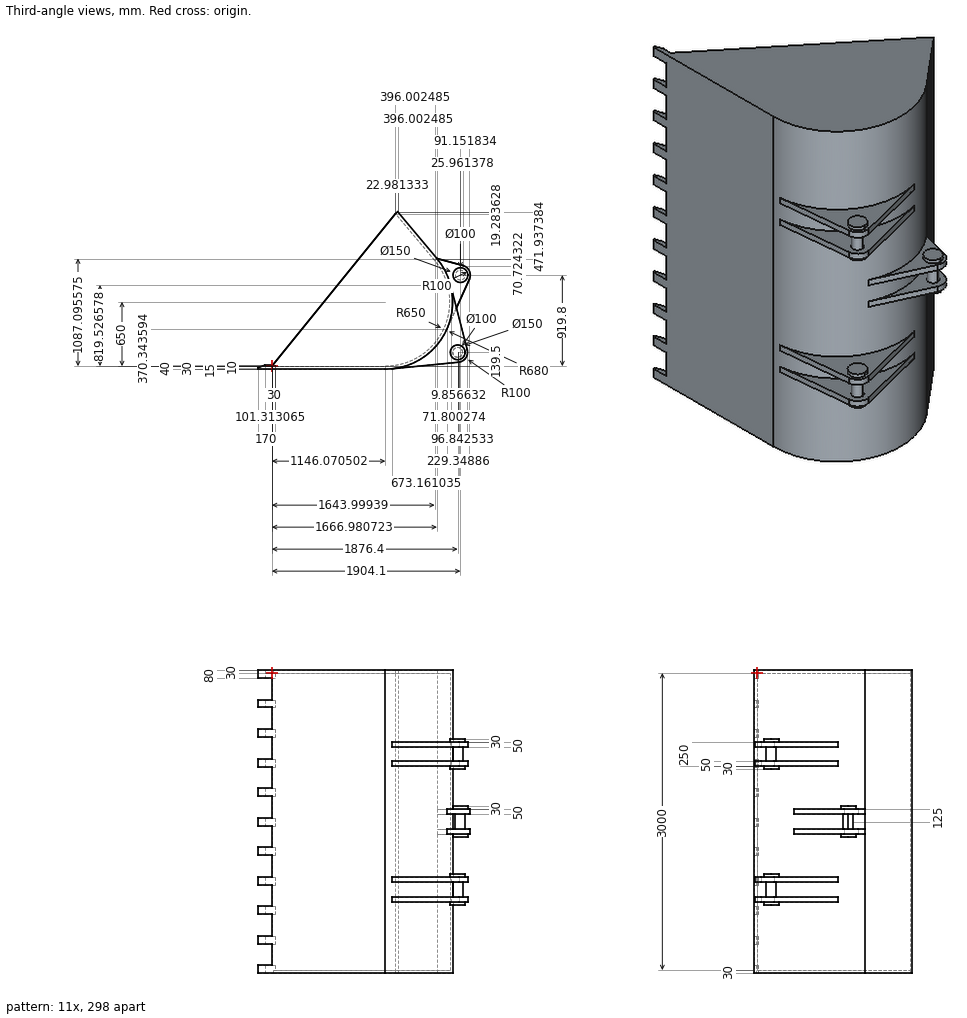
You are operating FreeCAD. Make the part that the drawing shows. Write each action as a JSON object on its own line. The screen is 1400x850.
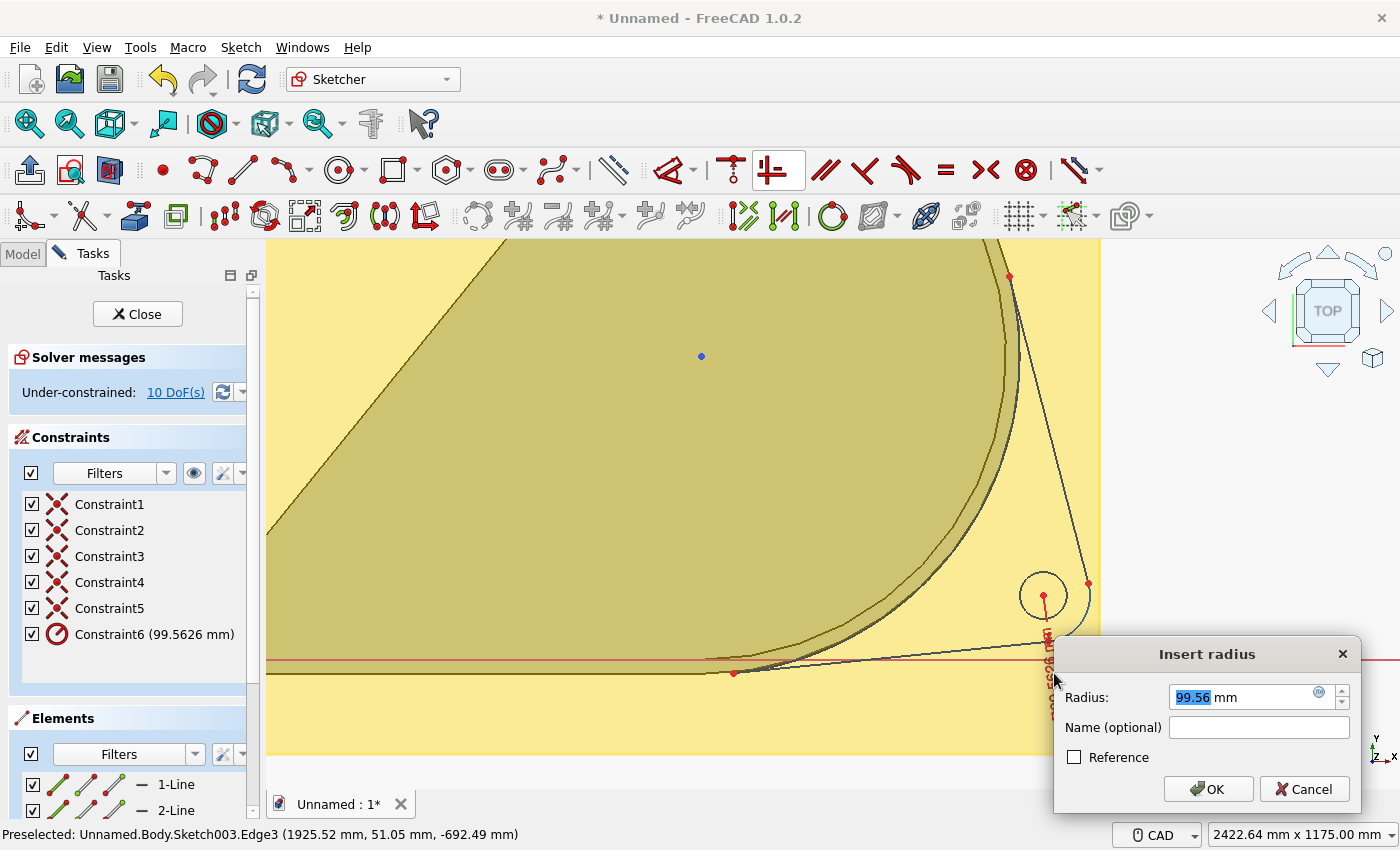
{"action": "type", "text": "100"}
{"action": "key", "text": "Return"}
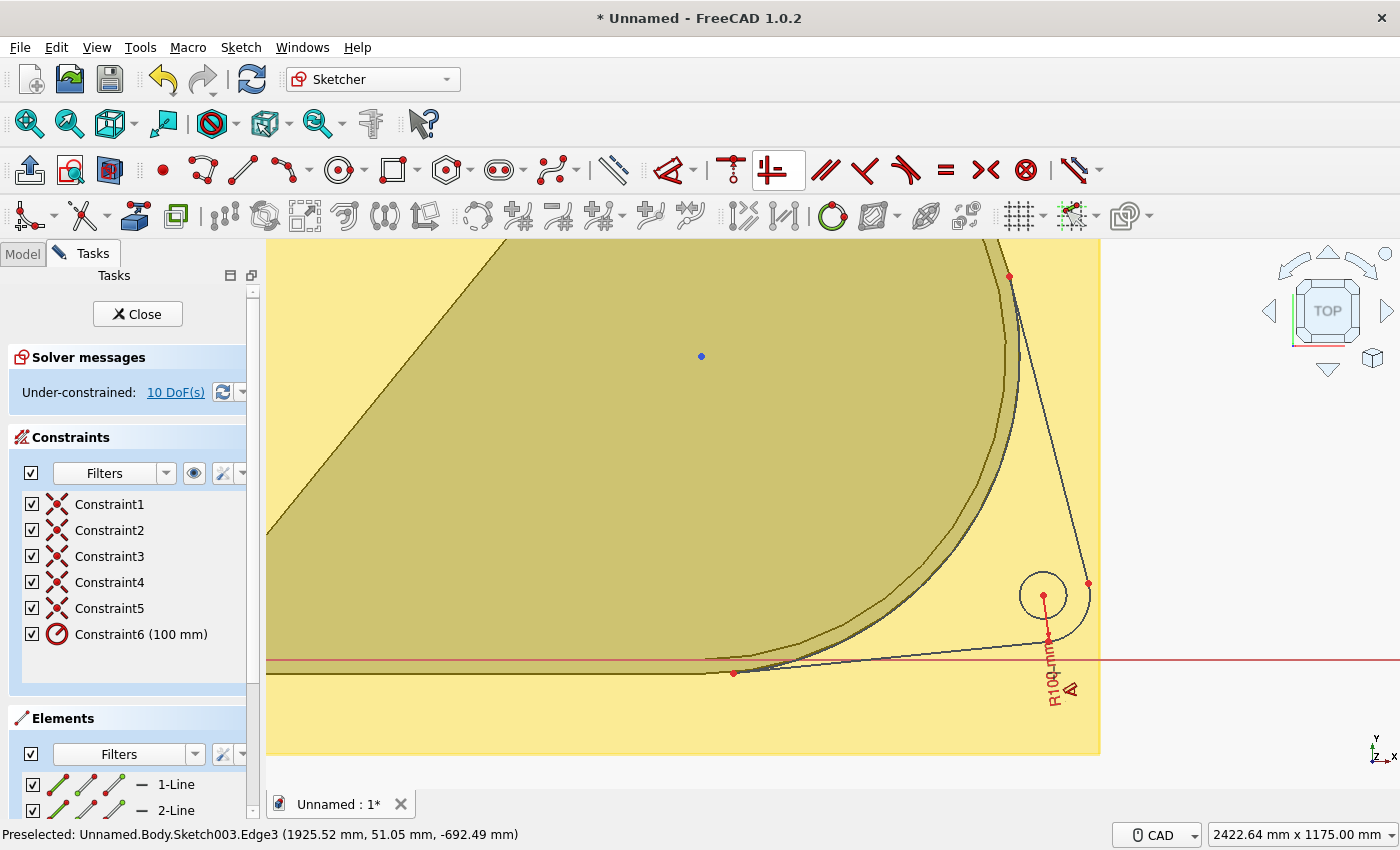
{"action": "left_click", "coordinate": [886, 616]}
{"action": "left_click", "coordinate": [905, 642]}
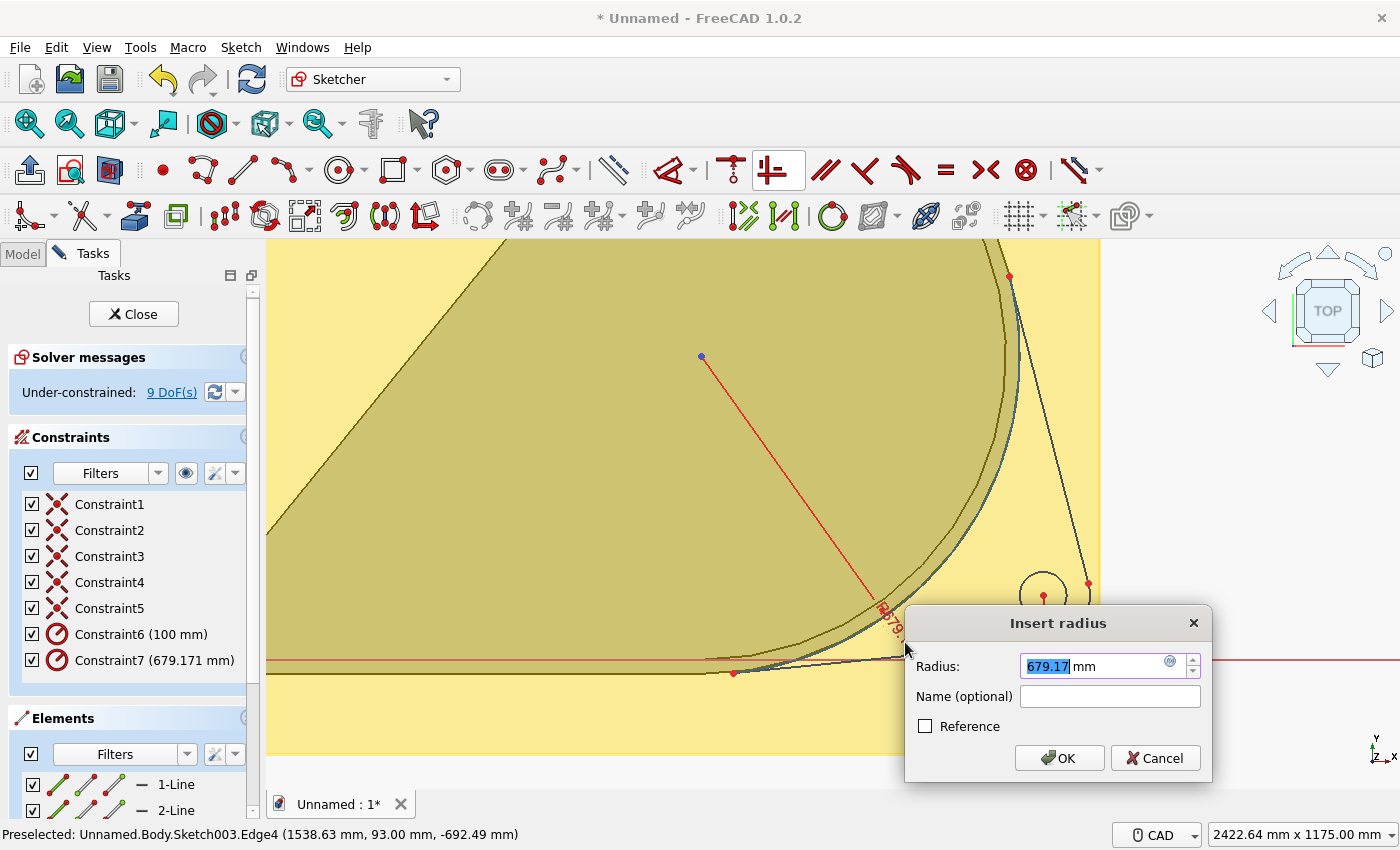
{"action": "type", "text": "680"}
{"action": "key", "text": "Return"}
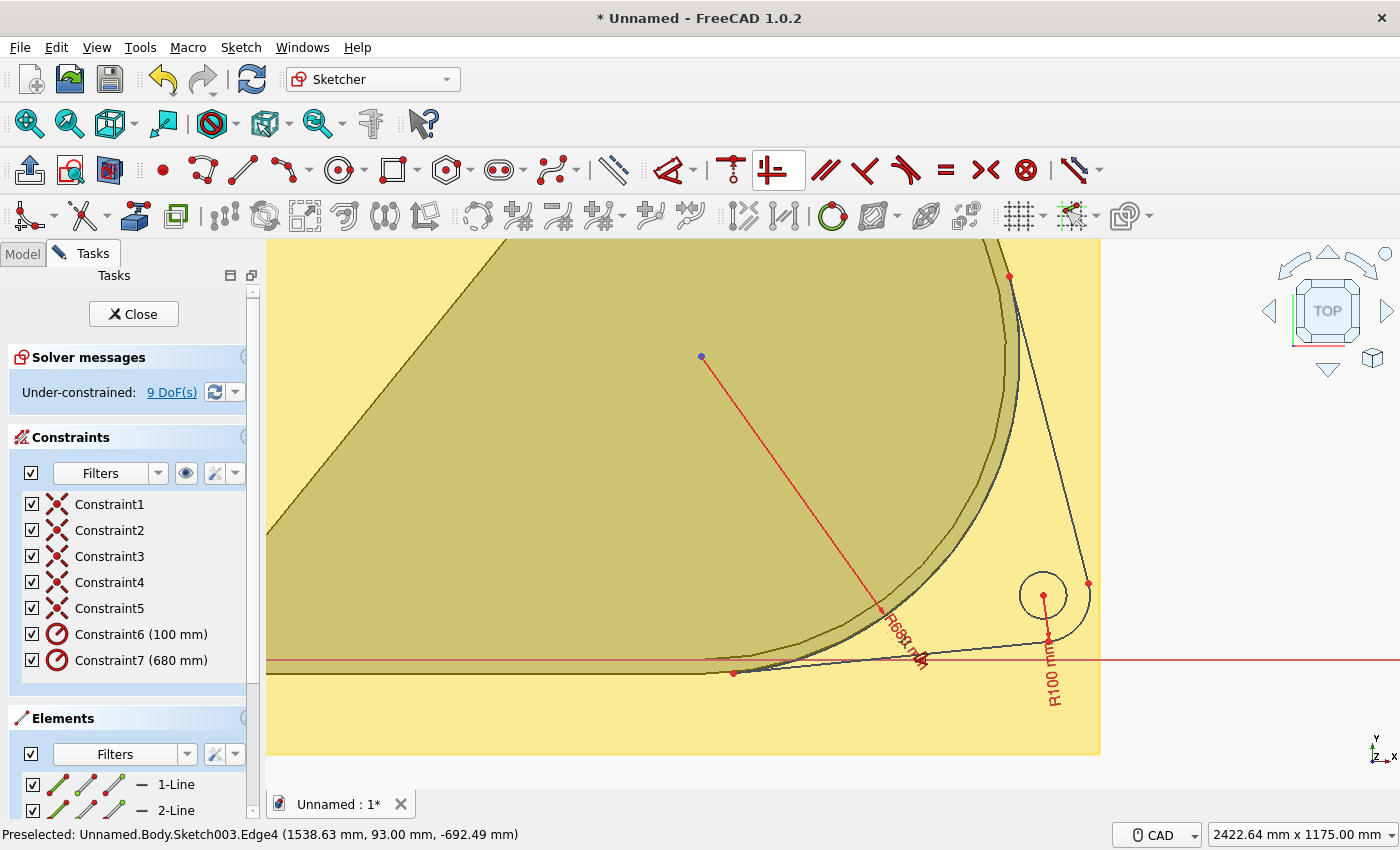
{"action": "left_click", "coordinate": [1060, 579]}
{"action": "left_click", "coordinate": [1060, 542]}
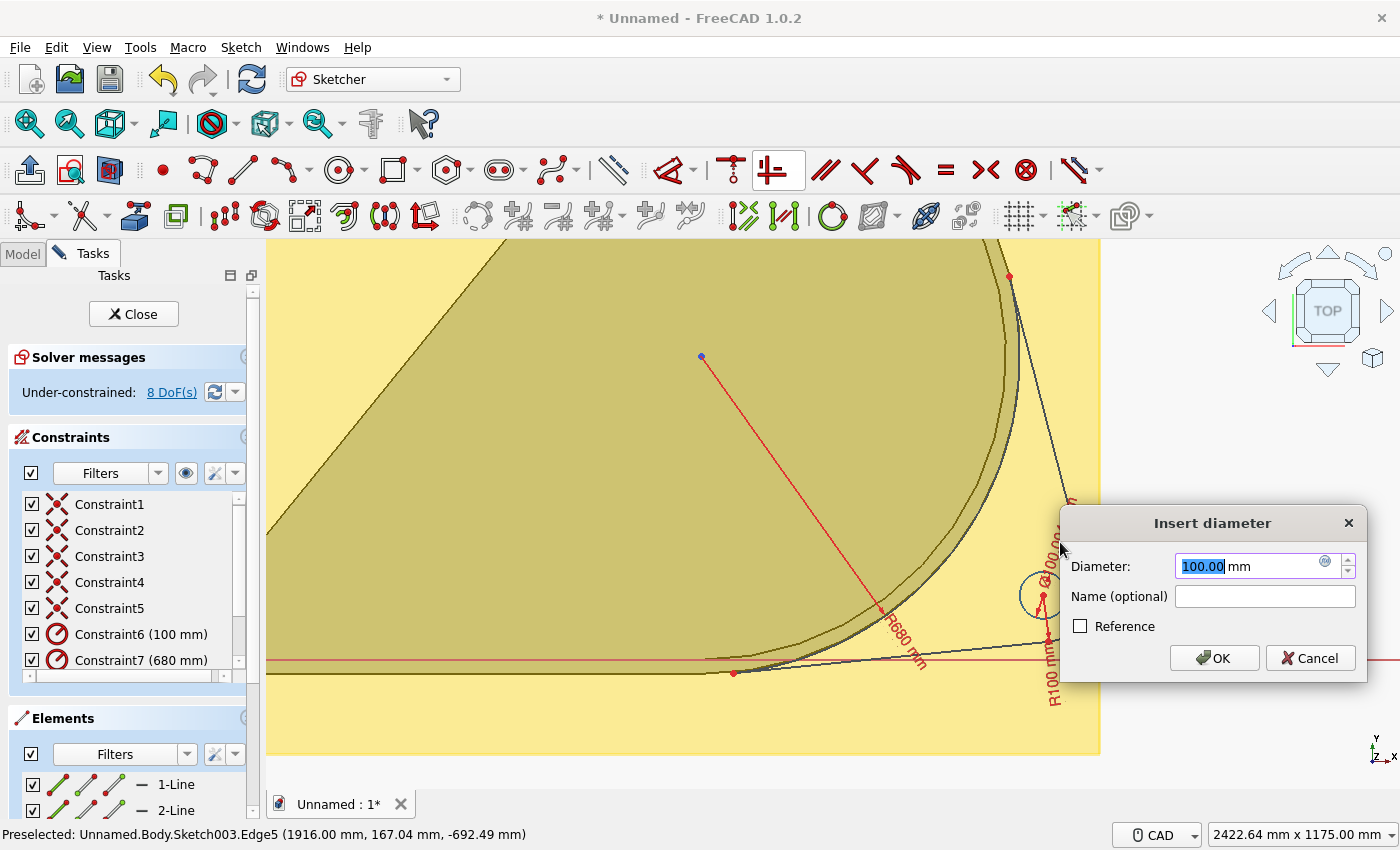
{"action": "type", "text": "100"}
{"action": "key", "text": "Return"}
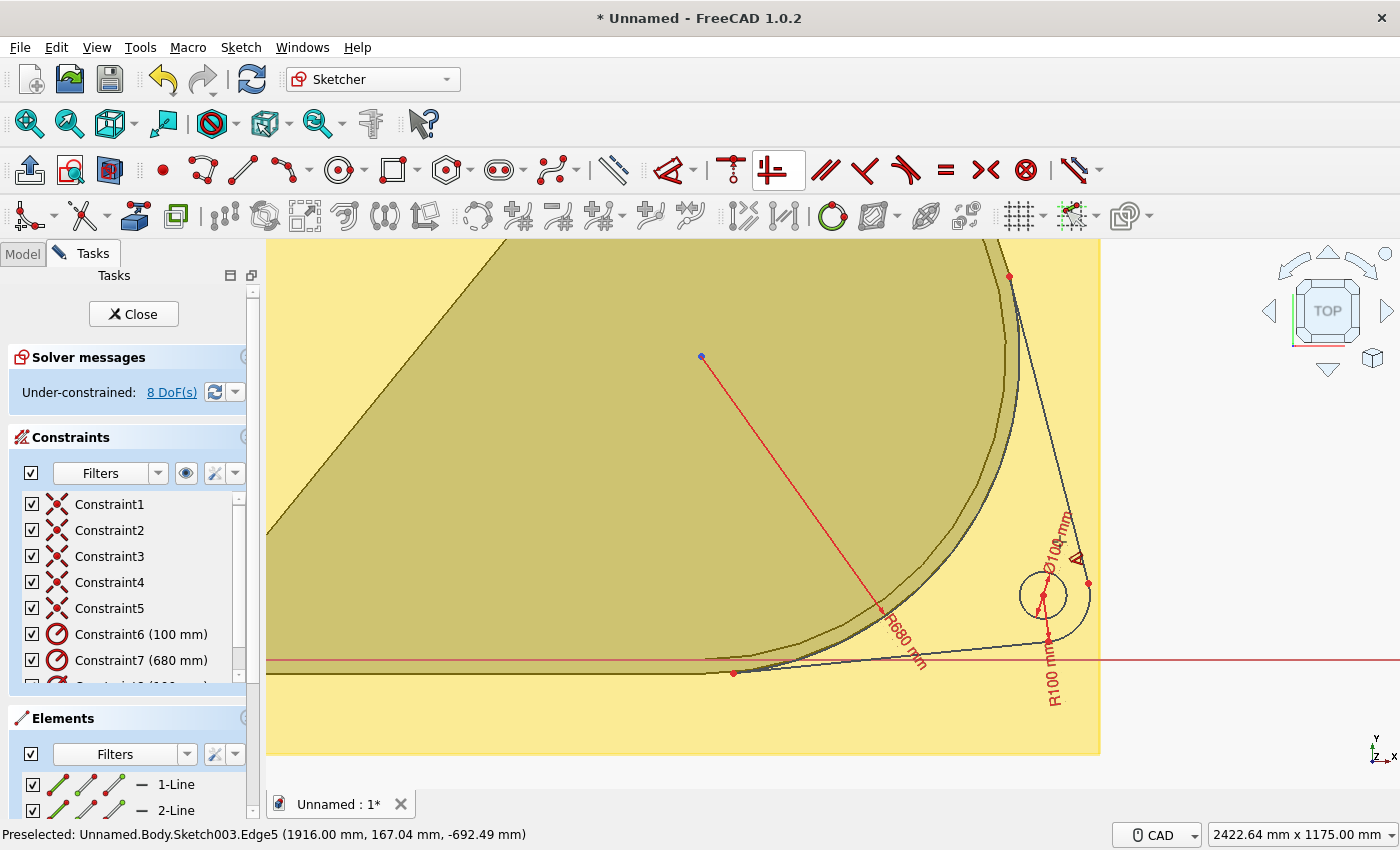
{"action": "left_click", "coordinate": [701, 357]}
{"action": "left_click", "coordinate": [735, 508]}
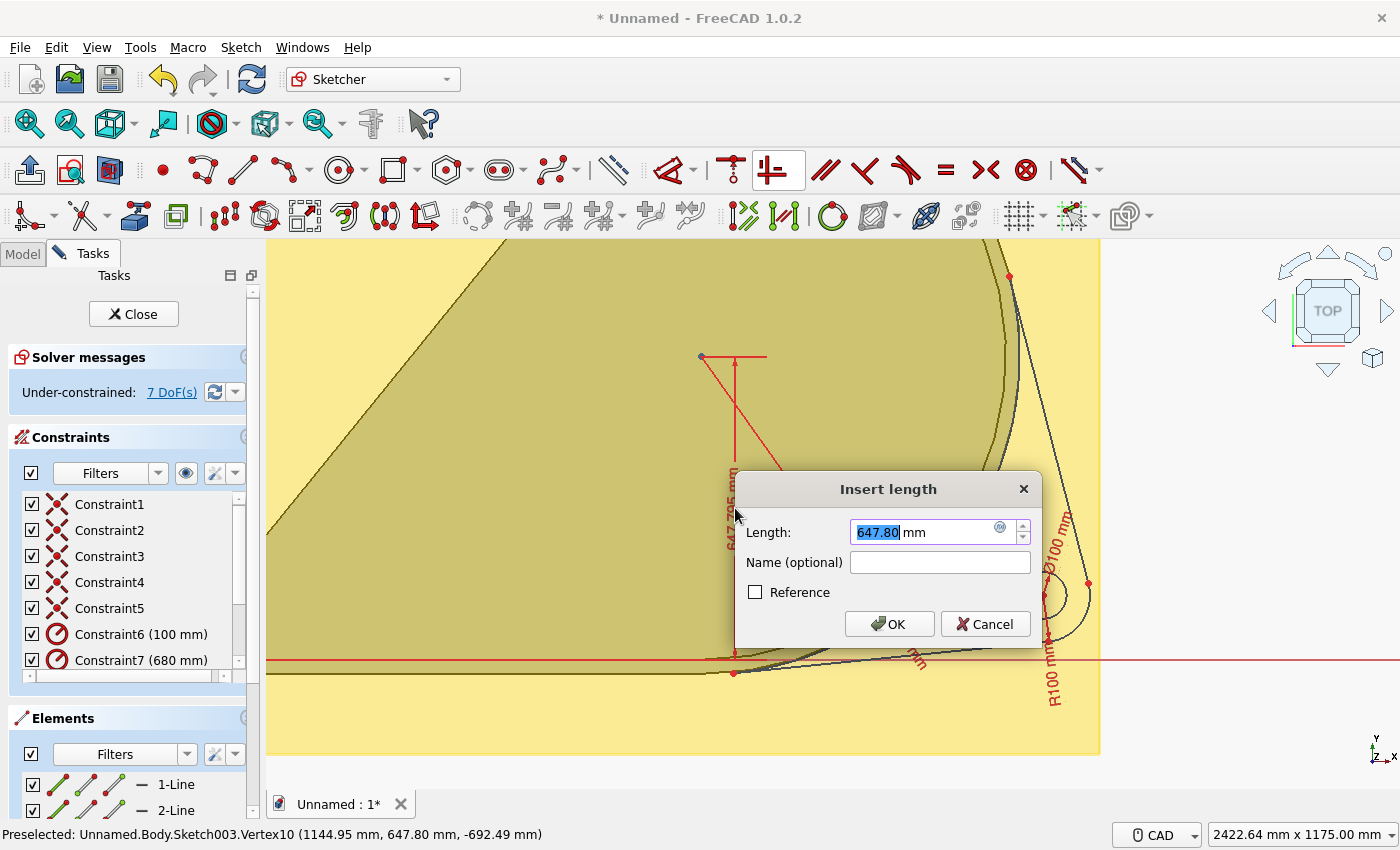
{"action": "type", "text": "650"}
{"action": "key", "text": "Return"}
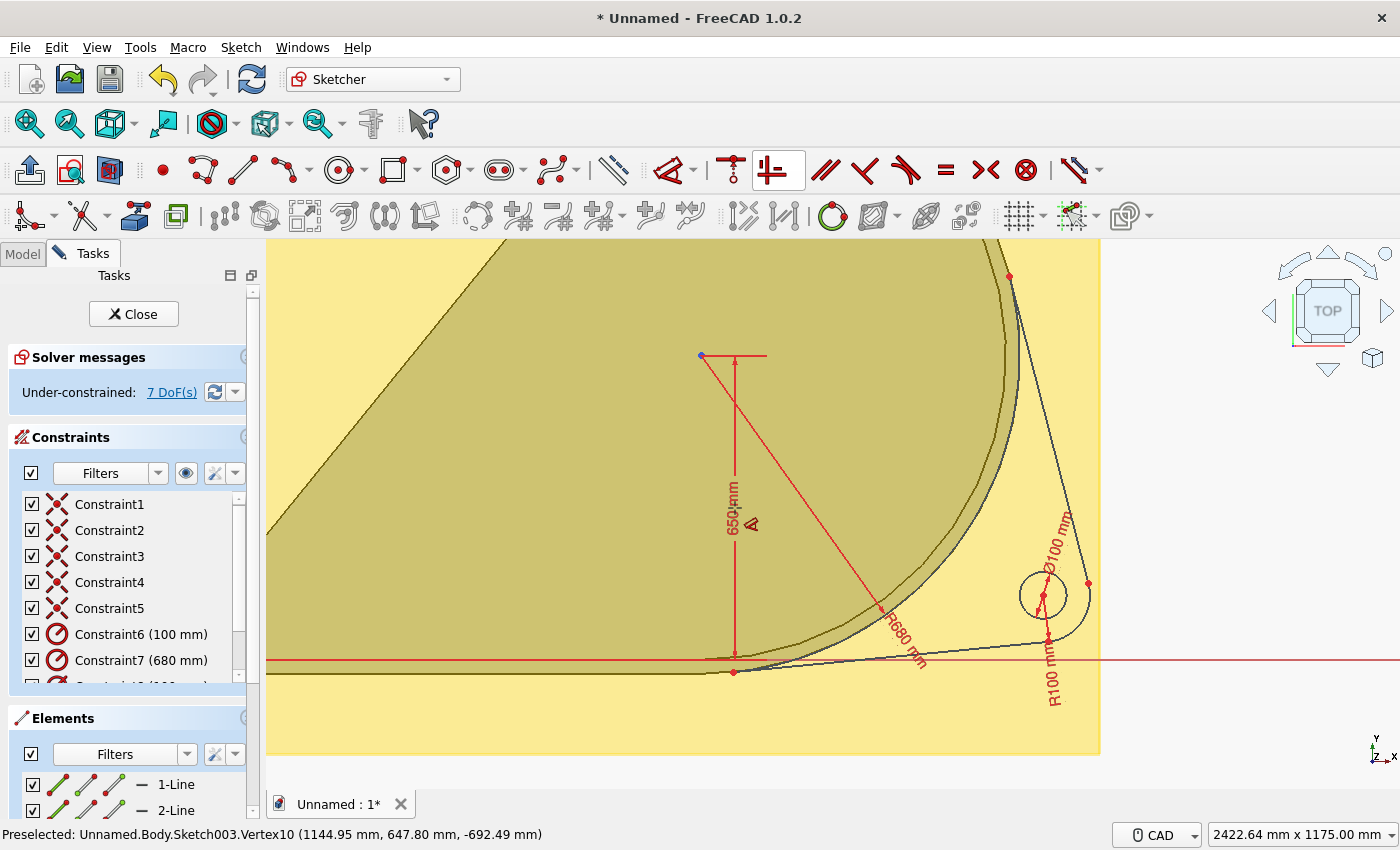
{"action": "left_click", "coordinate": [1043, 595]}
{"action": "left_click", "coordinate": [1101, 628]}